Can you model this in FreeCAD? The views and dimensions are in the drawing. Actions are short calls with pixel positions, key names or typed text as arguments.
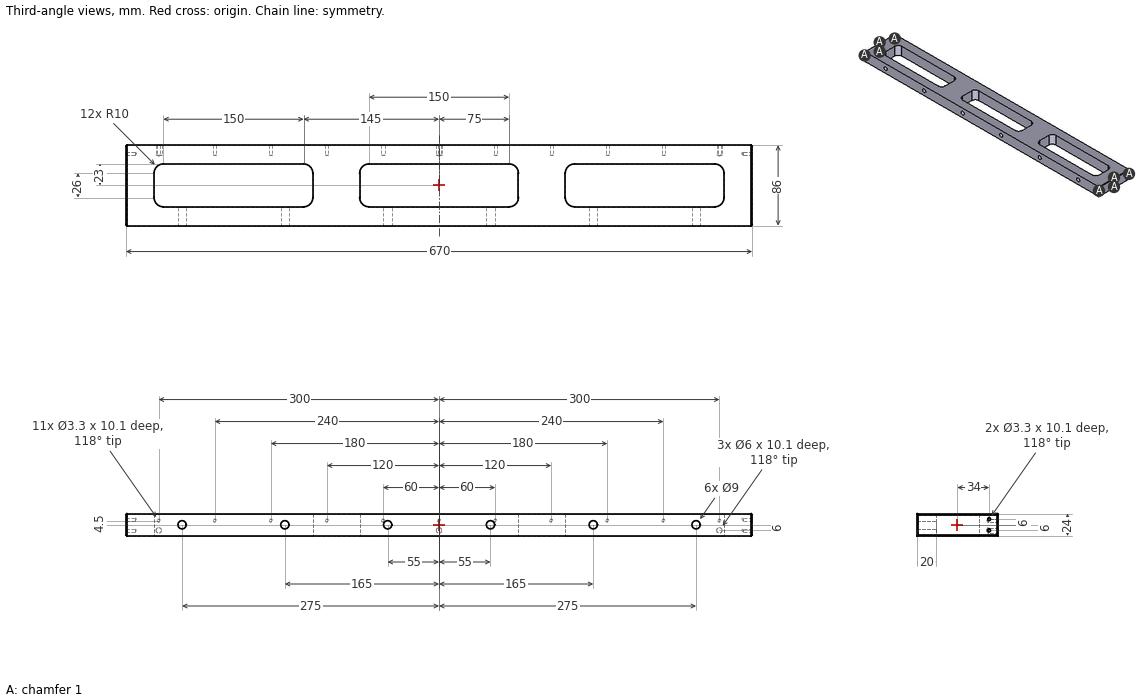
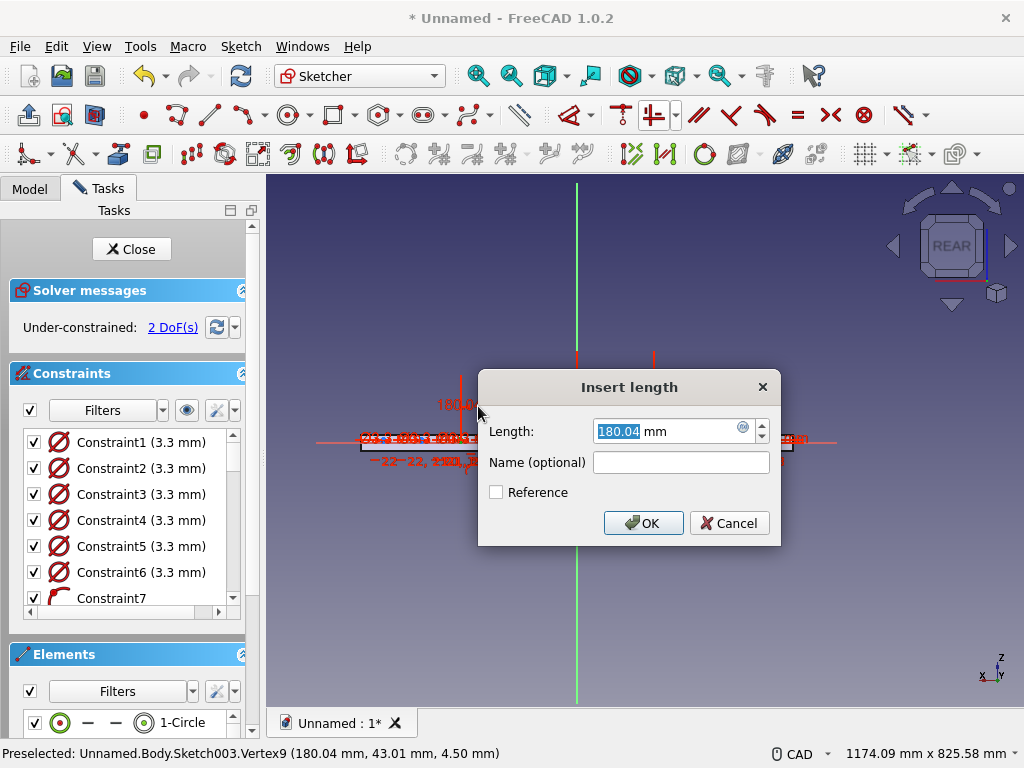
text(180)
key(Return)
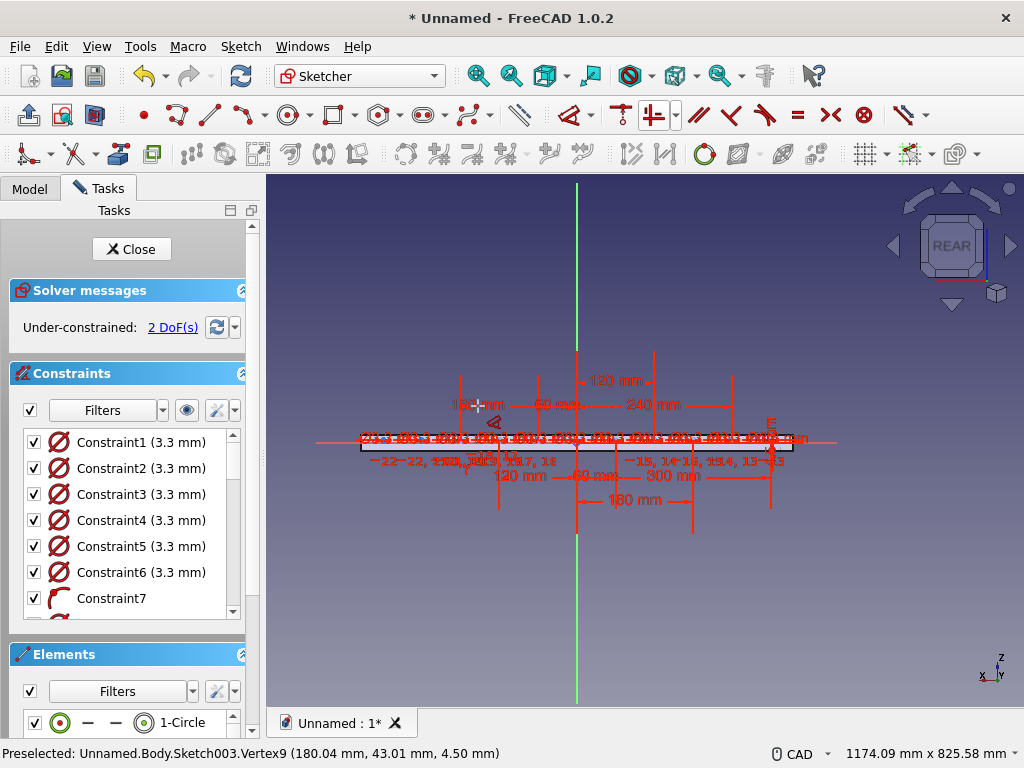
click(422, 440)
click(445, 477)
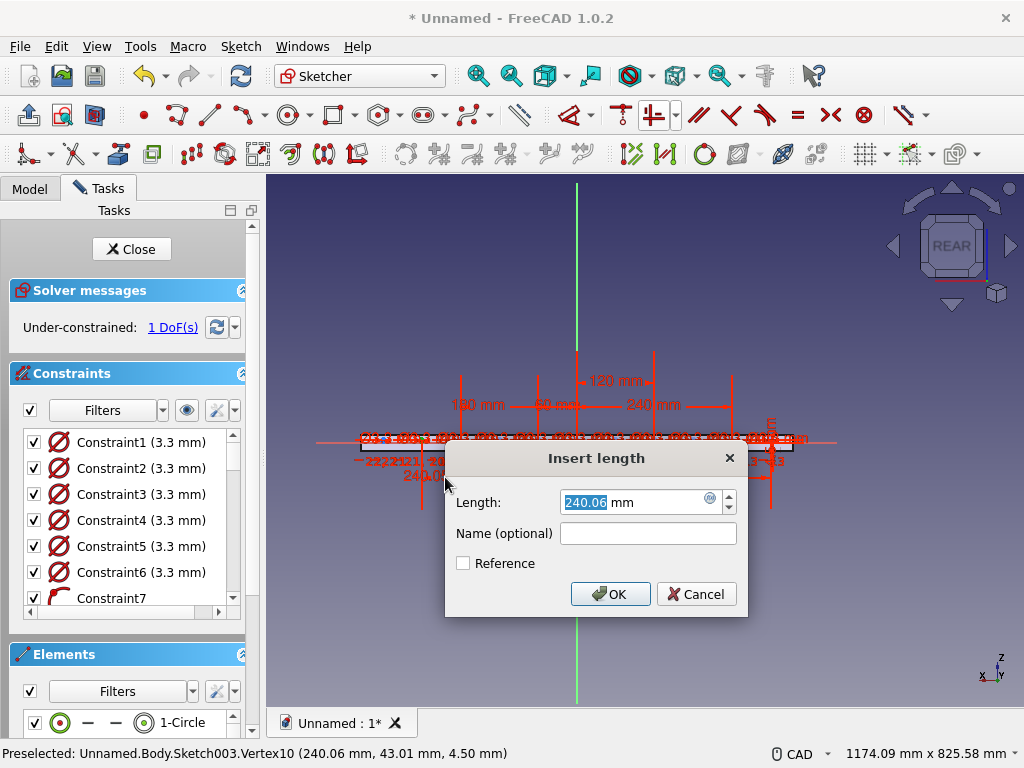
text(240)
key(Return)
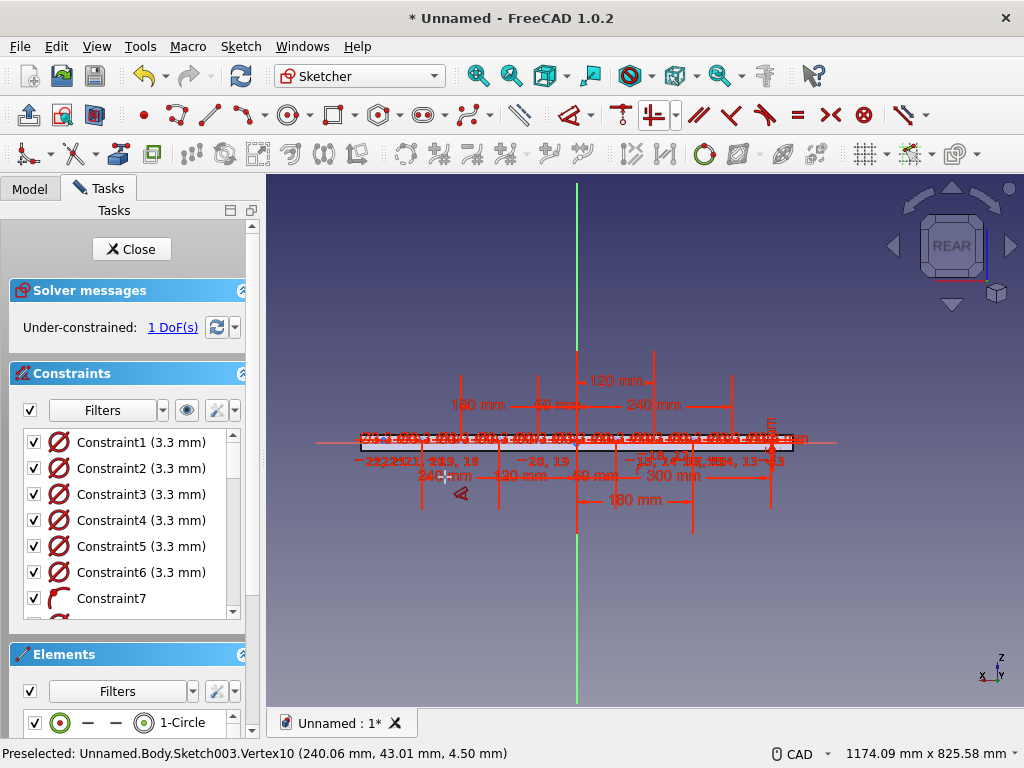
click(383, 440)
click(480, 501)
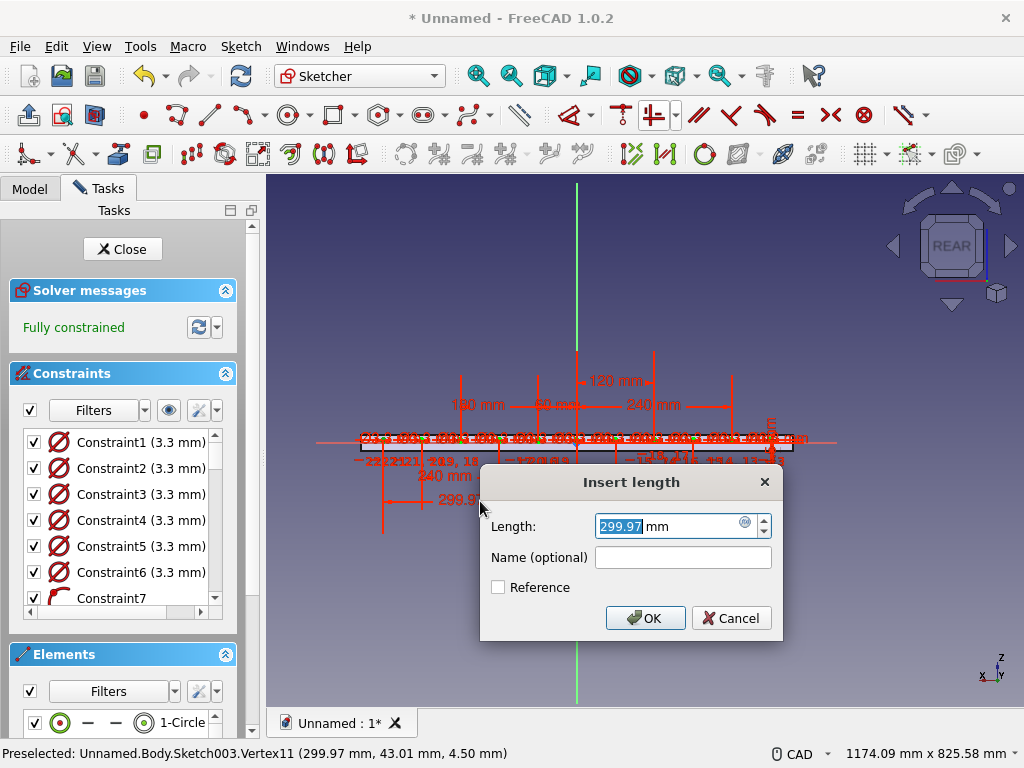
text(300)
key(Return)
key(Escape)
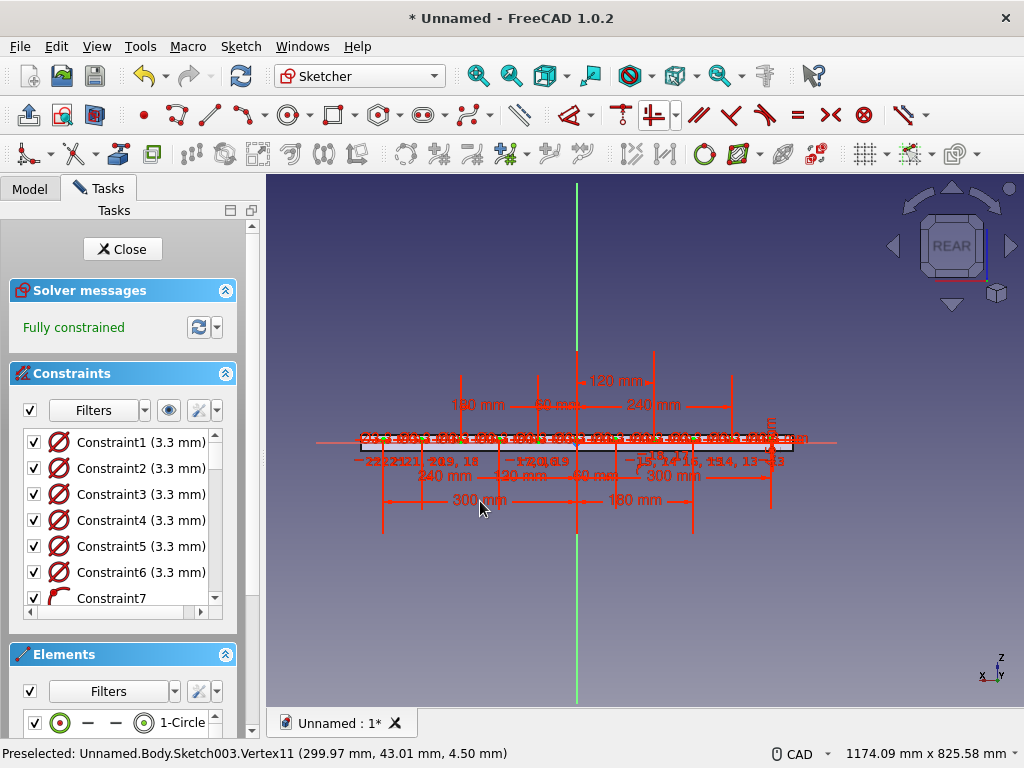
click(123, 249)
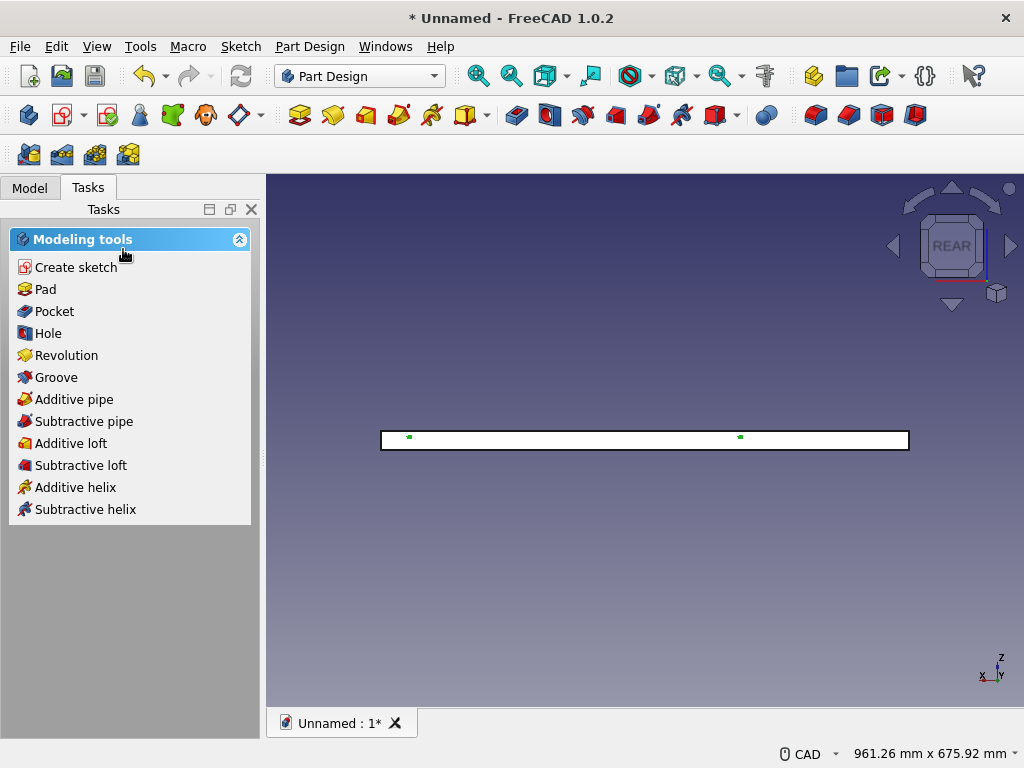
click(550, 116)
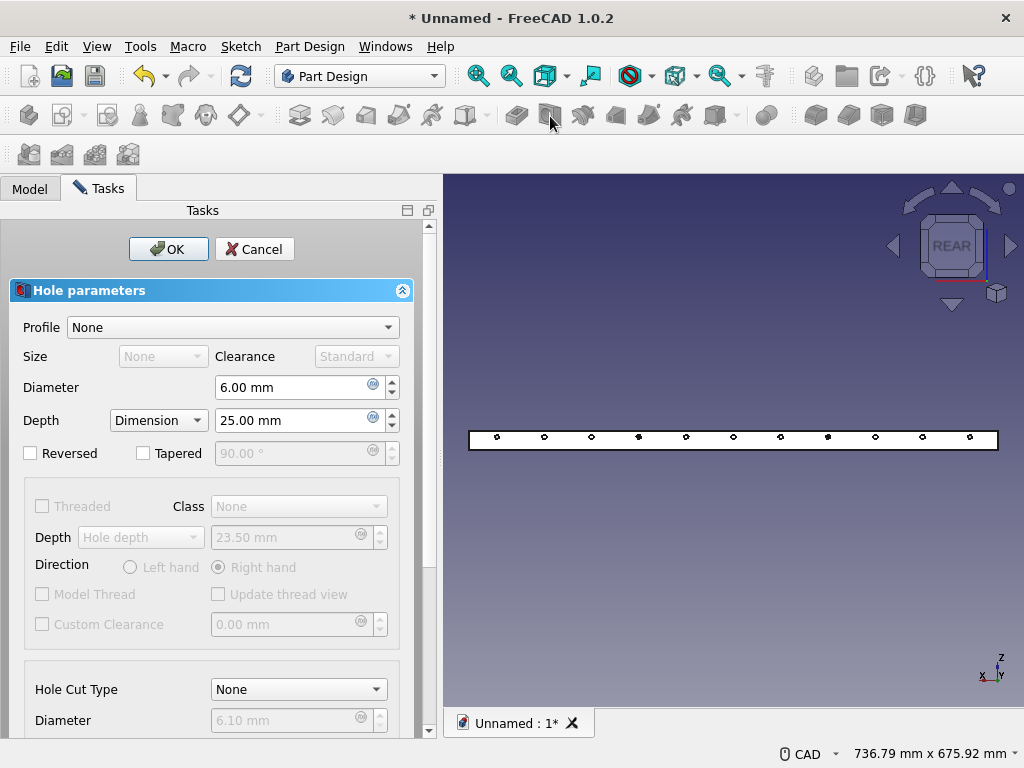
triple_click(300, 388)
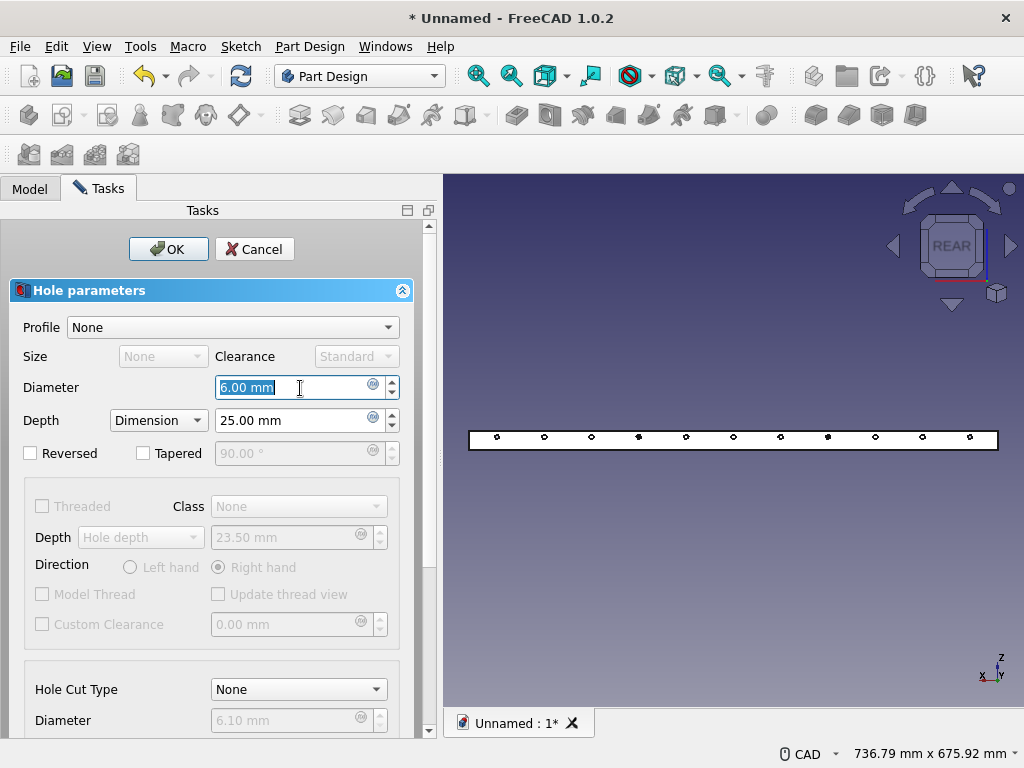
text(3.3)
key(Tab)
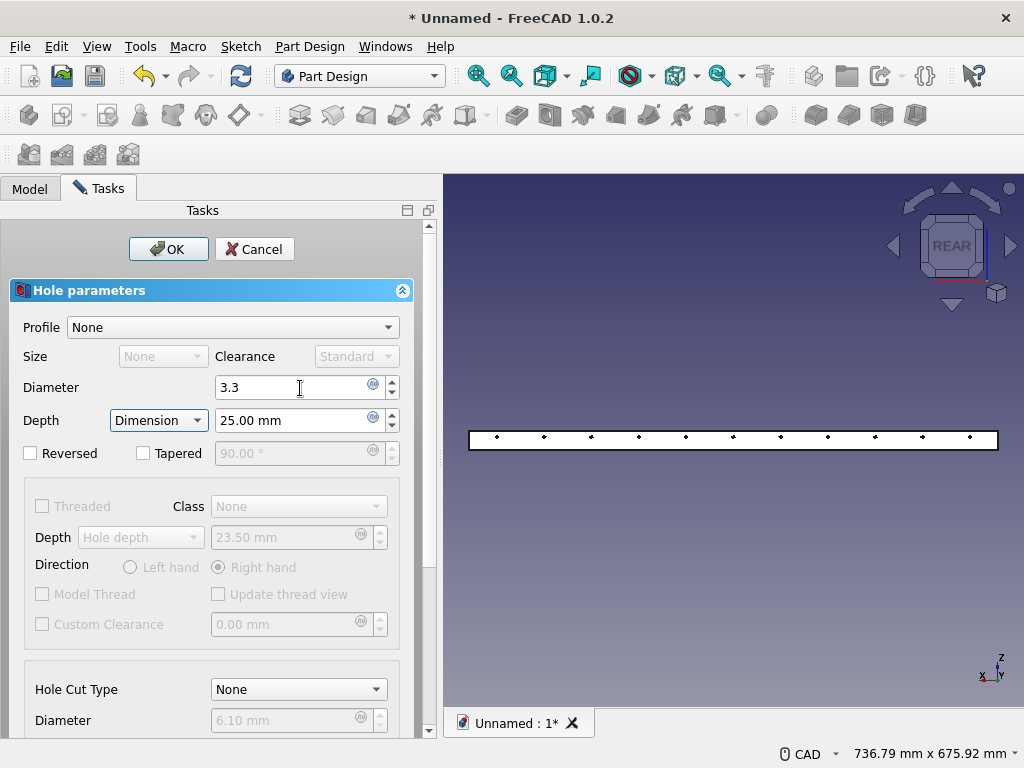
triple_click(300, 420)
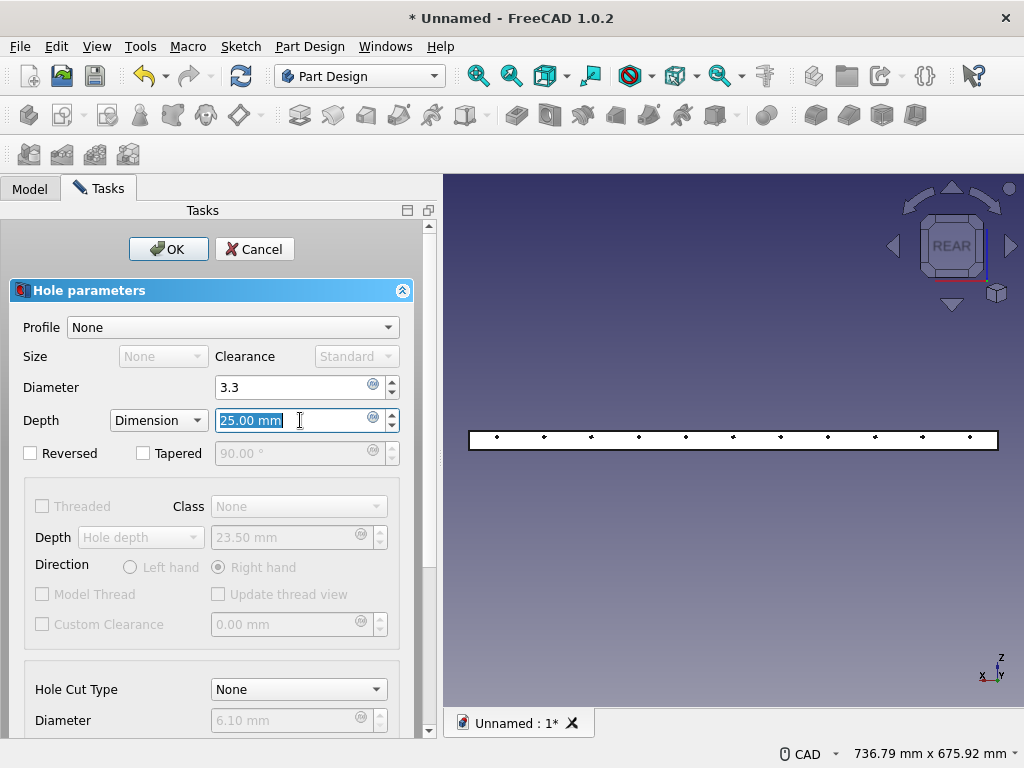
text(10.1)
key(Tab)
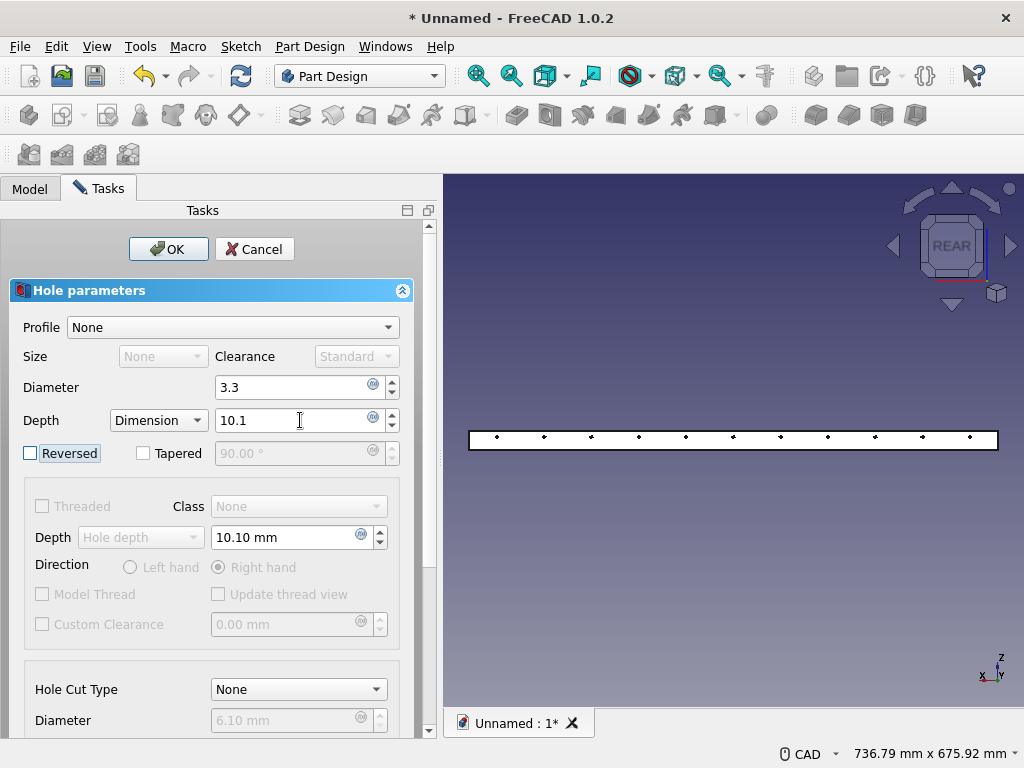
click(169, 249)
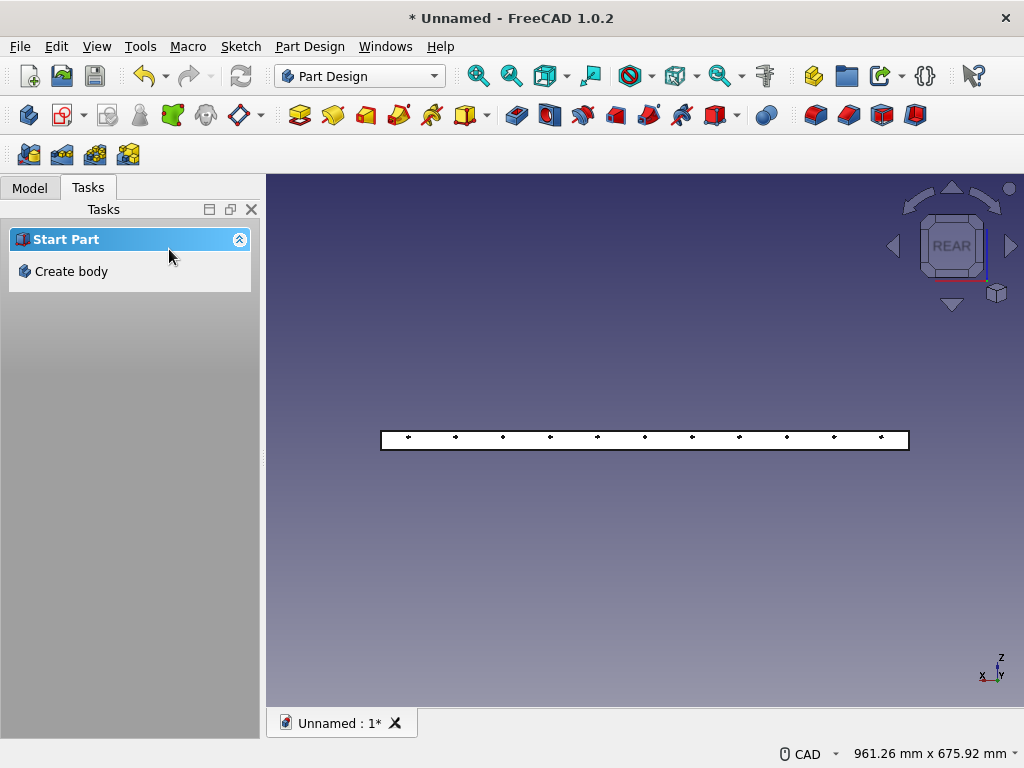
click(570, 439)